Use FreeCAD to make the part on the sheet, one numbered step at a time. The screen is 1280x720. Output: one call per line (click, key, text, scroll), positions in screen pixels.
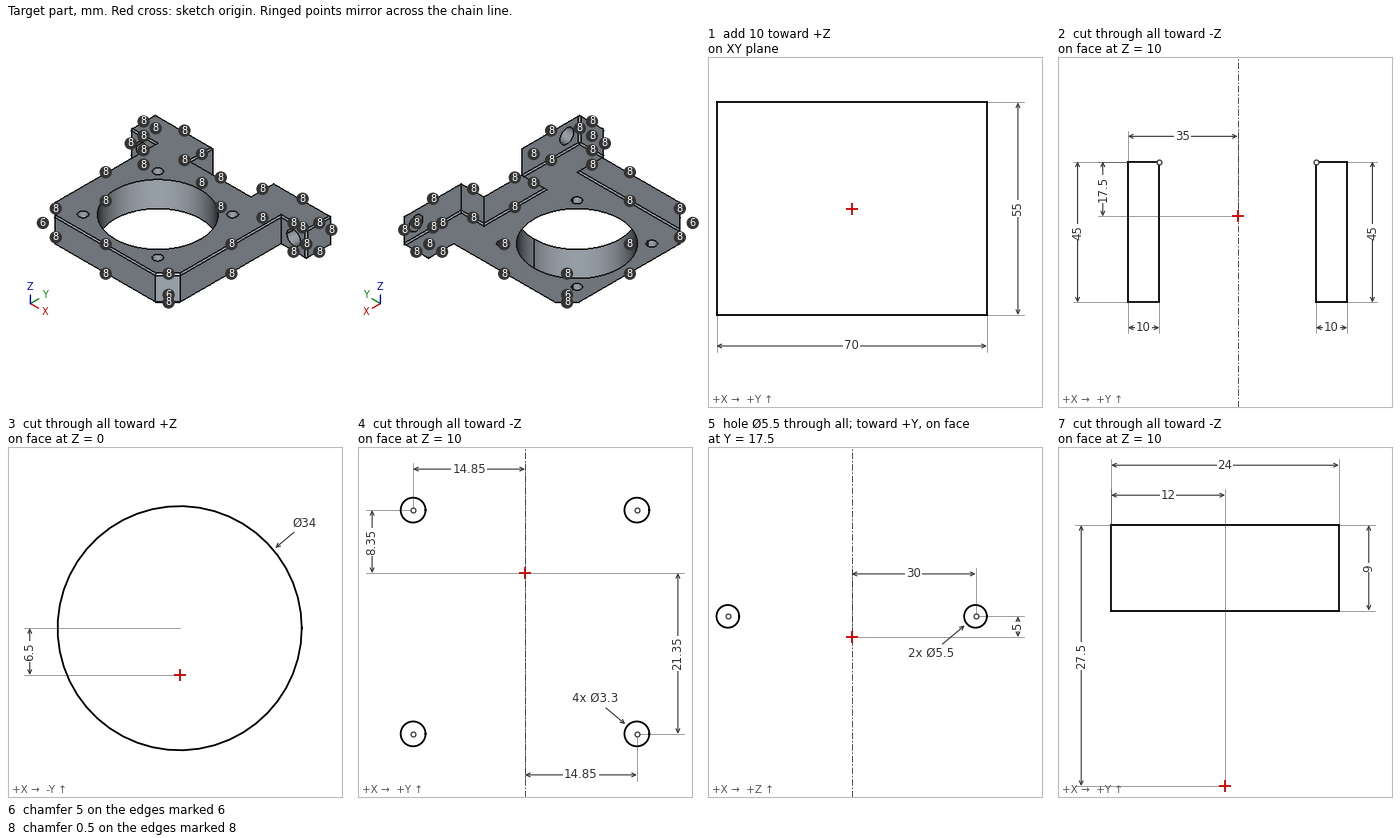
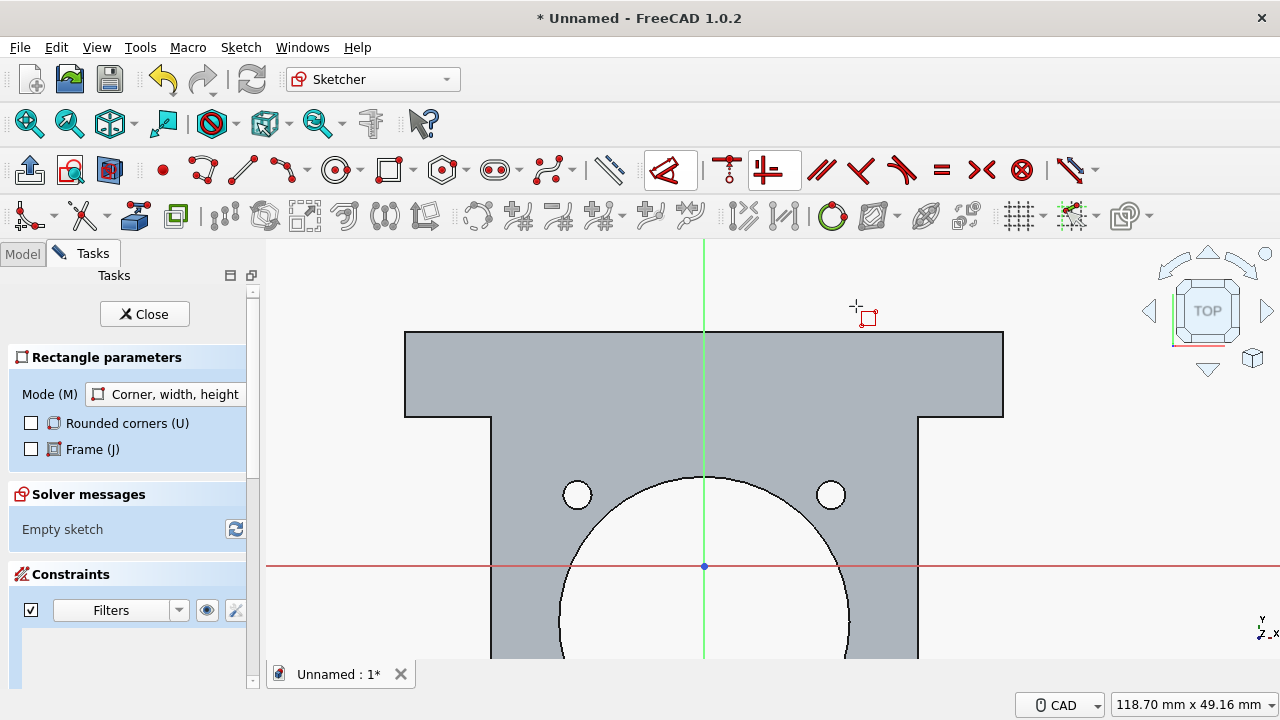
click(602, 332)
move(807, 408)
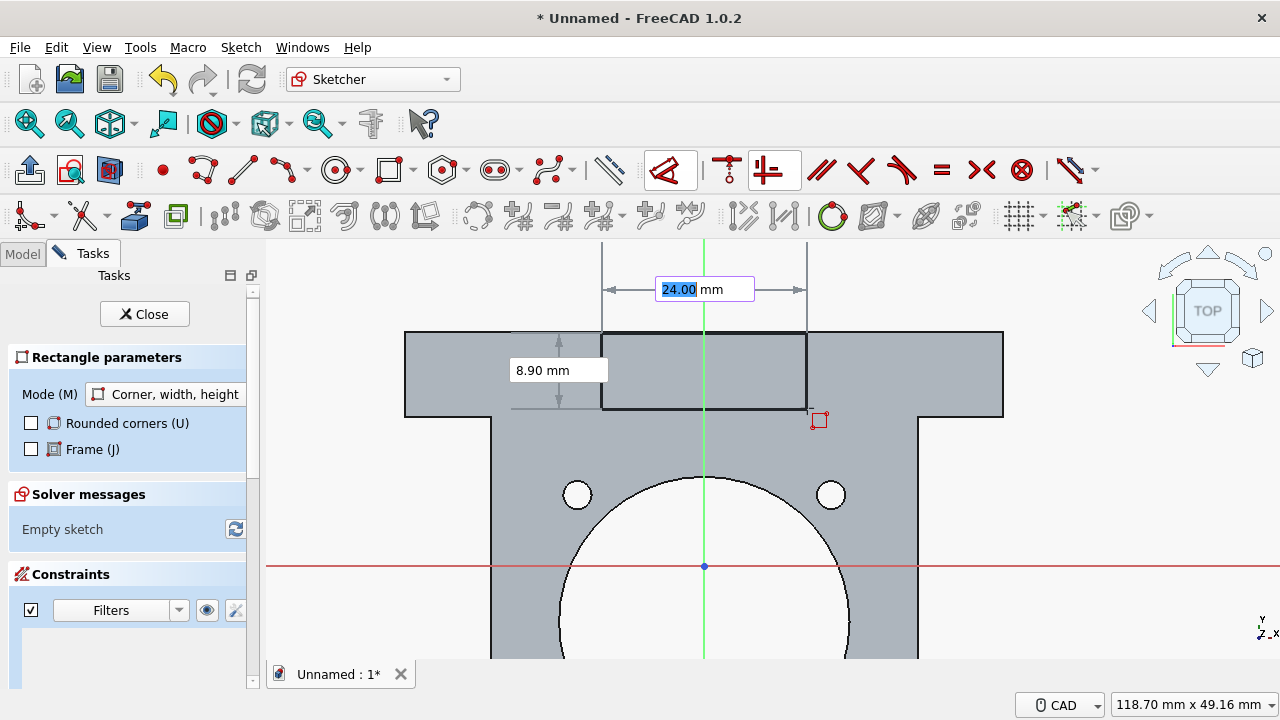
text(24)
key(Tab)
text(9)
key(Return)
key(Escape)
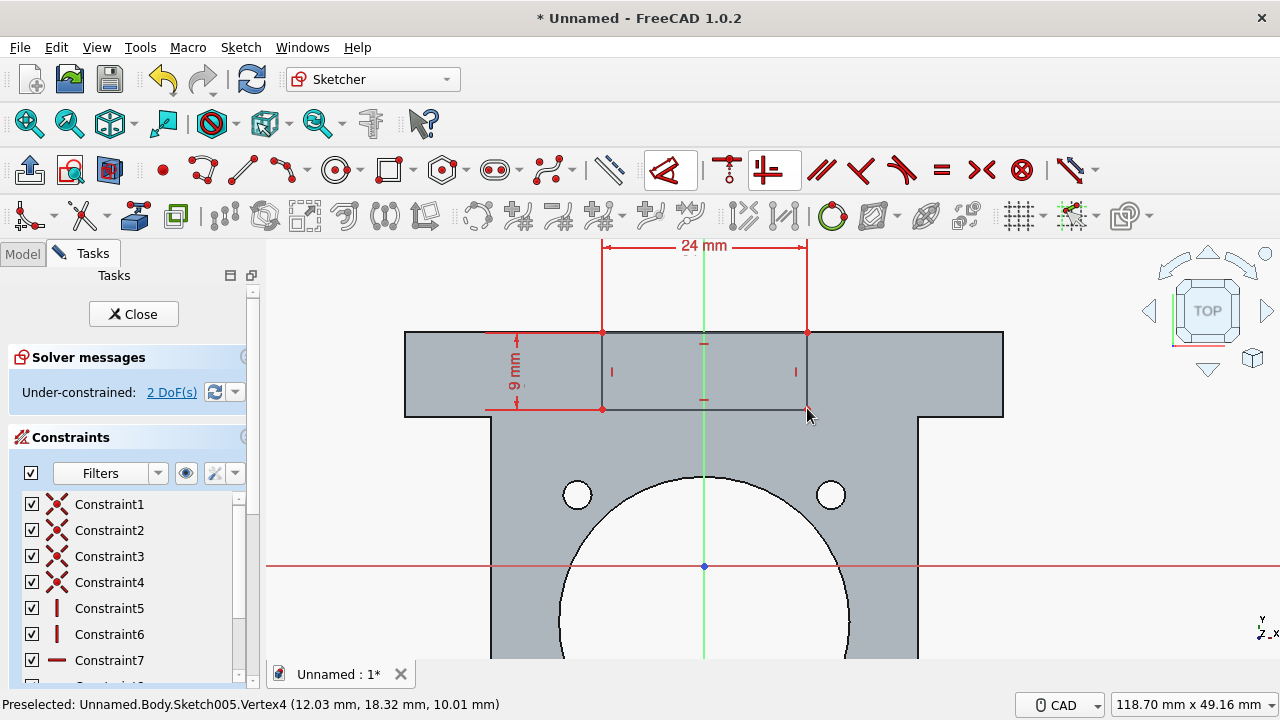
click(602, 333)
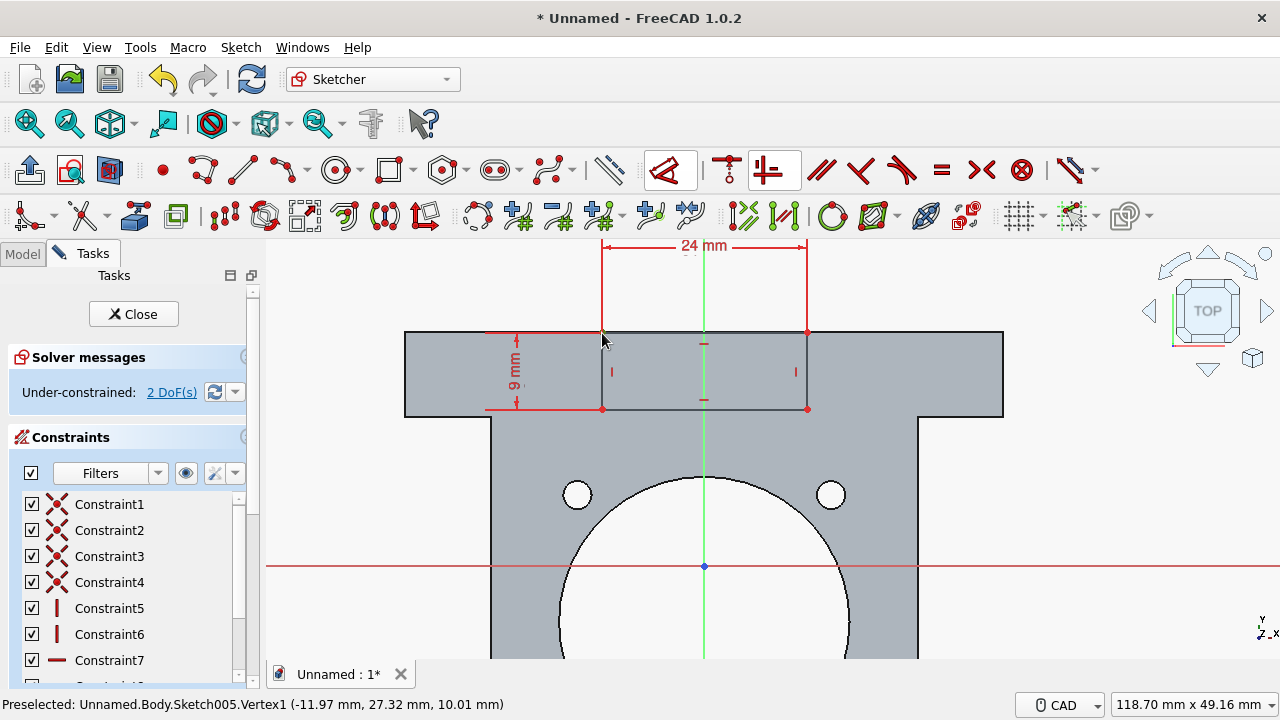
key(l)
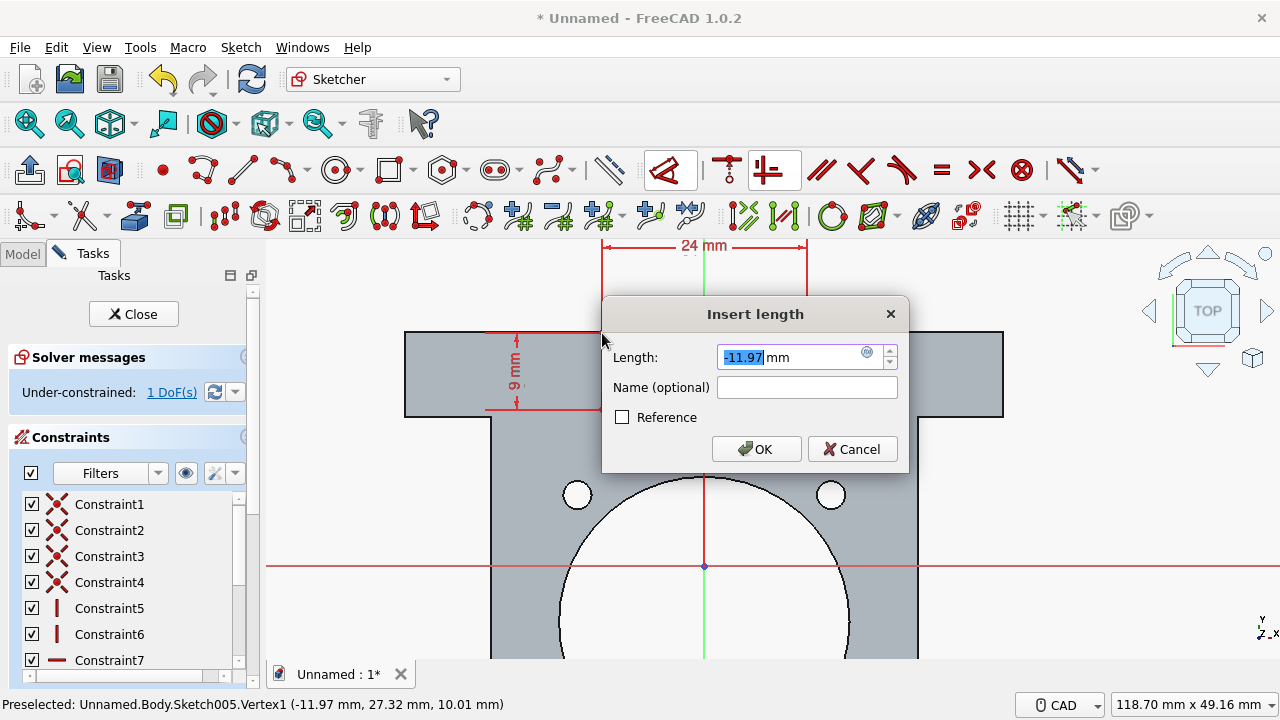
text(-12)
key(Return)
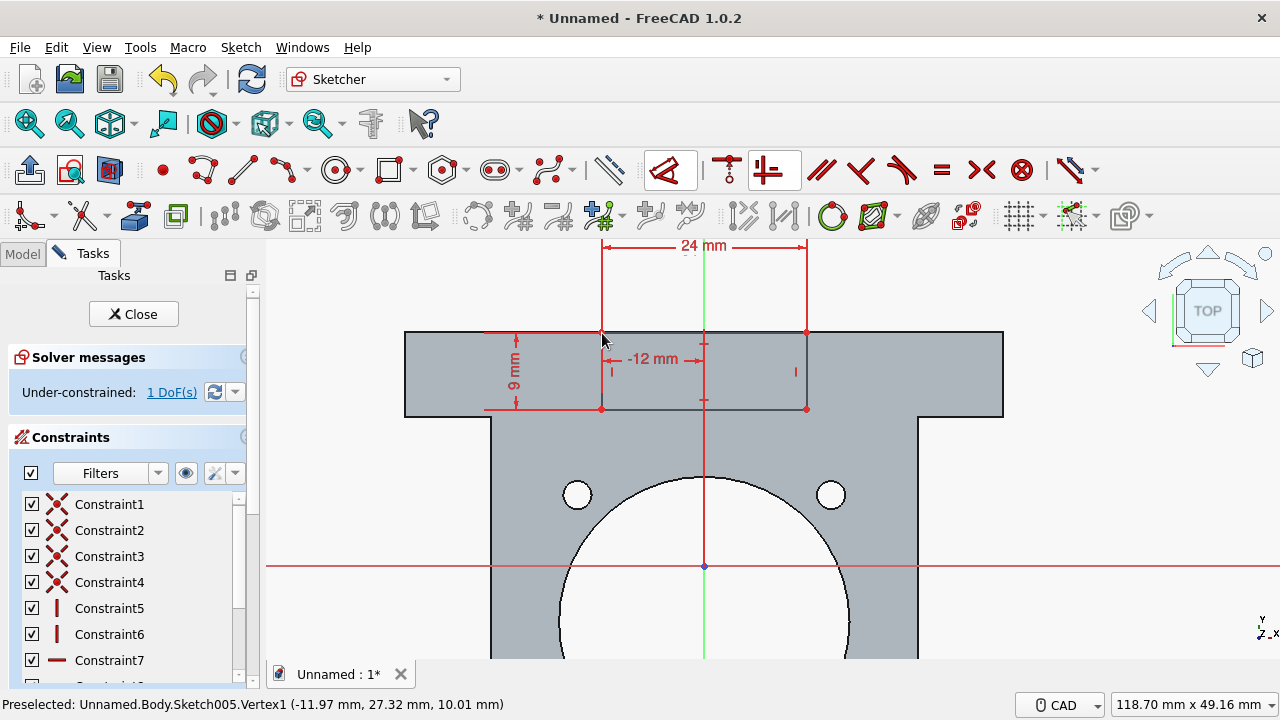
click(602, 333)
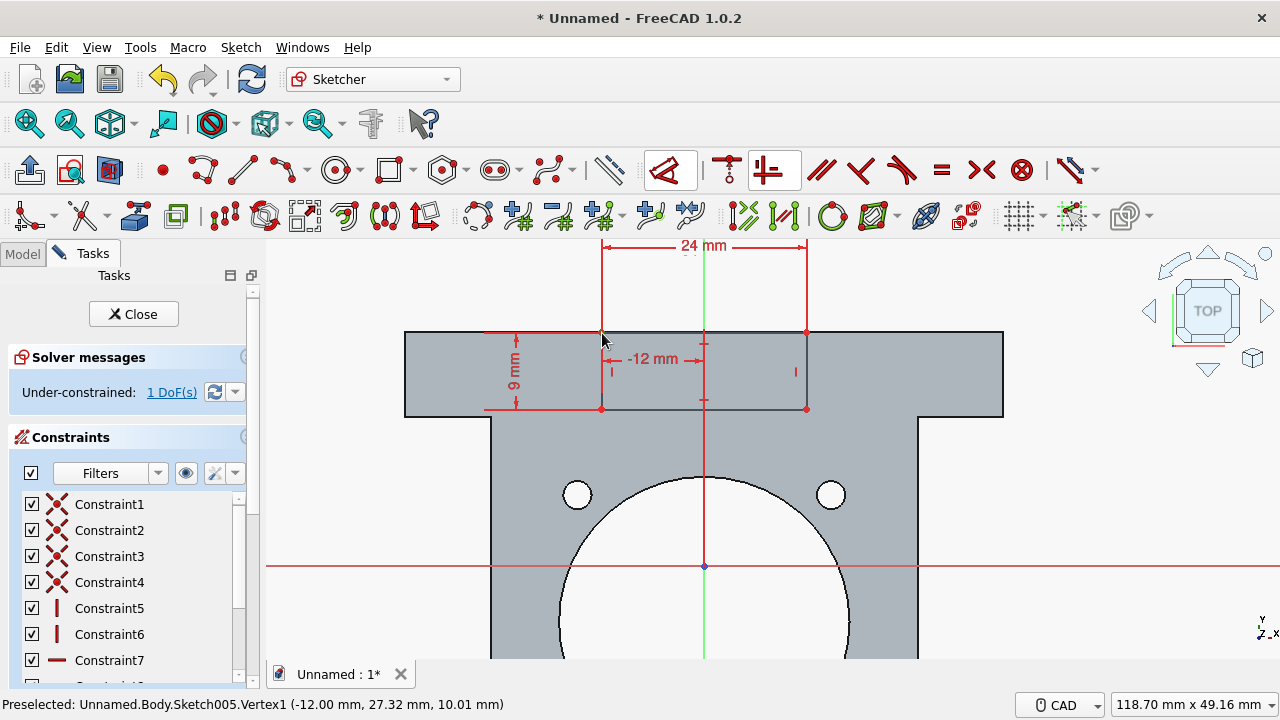
click(692, 170)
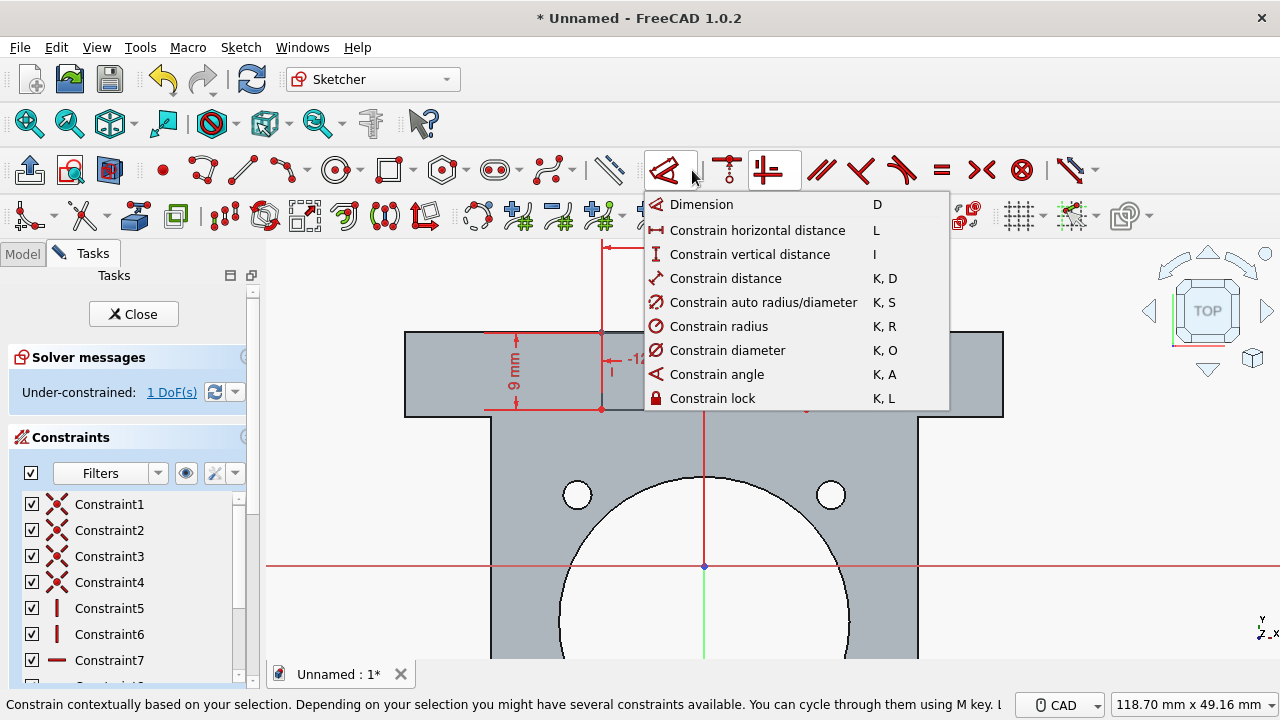
click(797, 254)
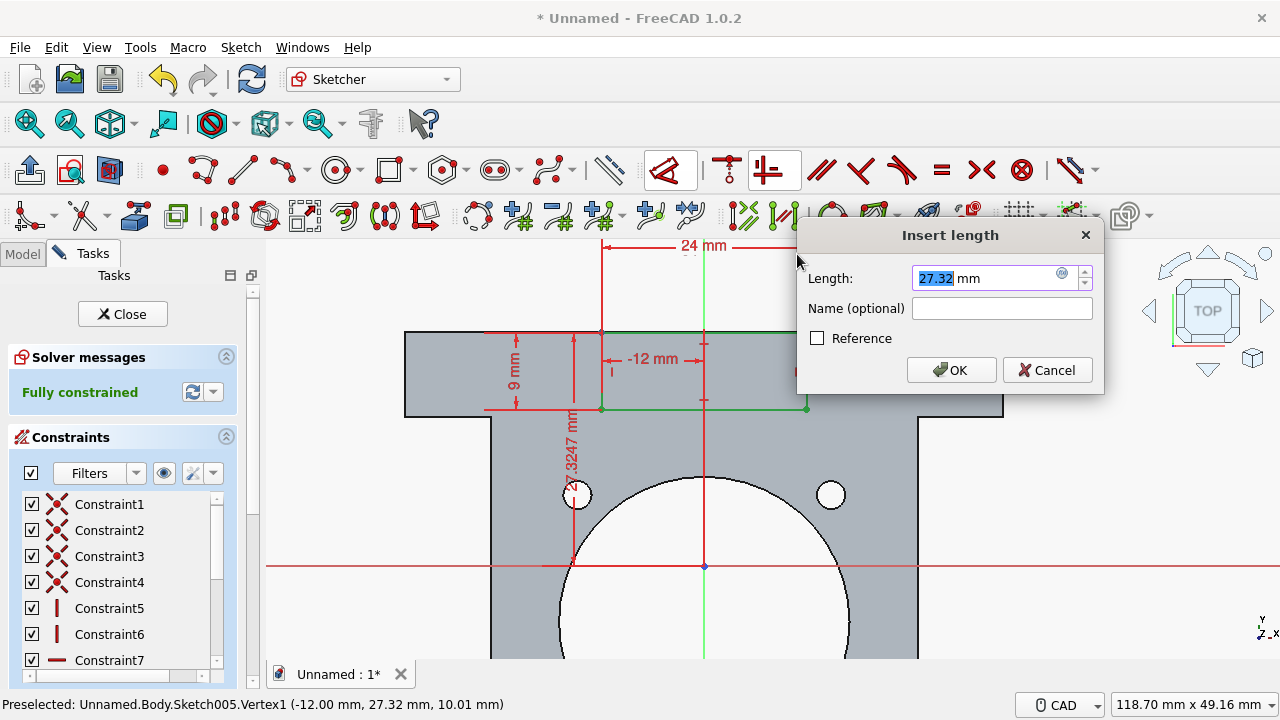
text(27.5)
key(Return)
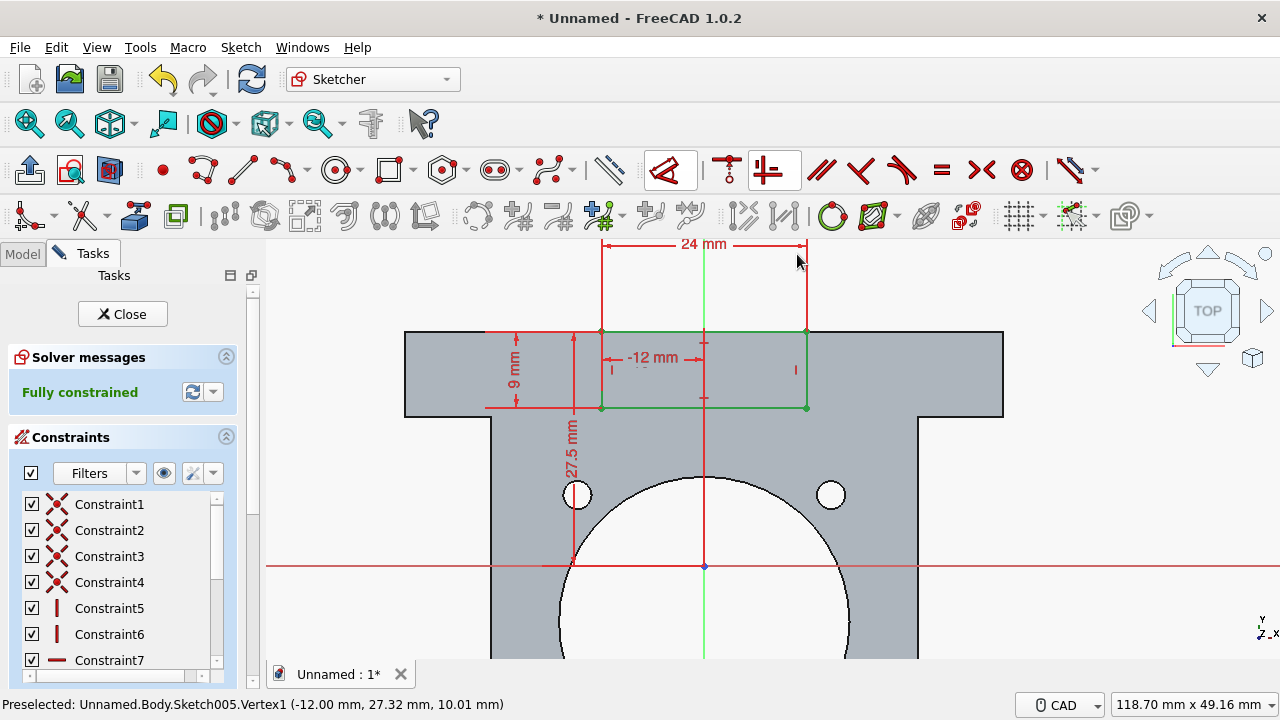
click(123, 314)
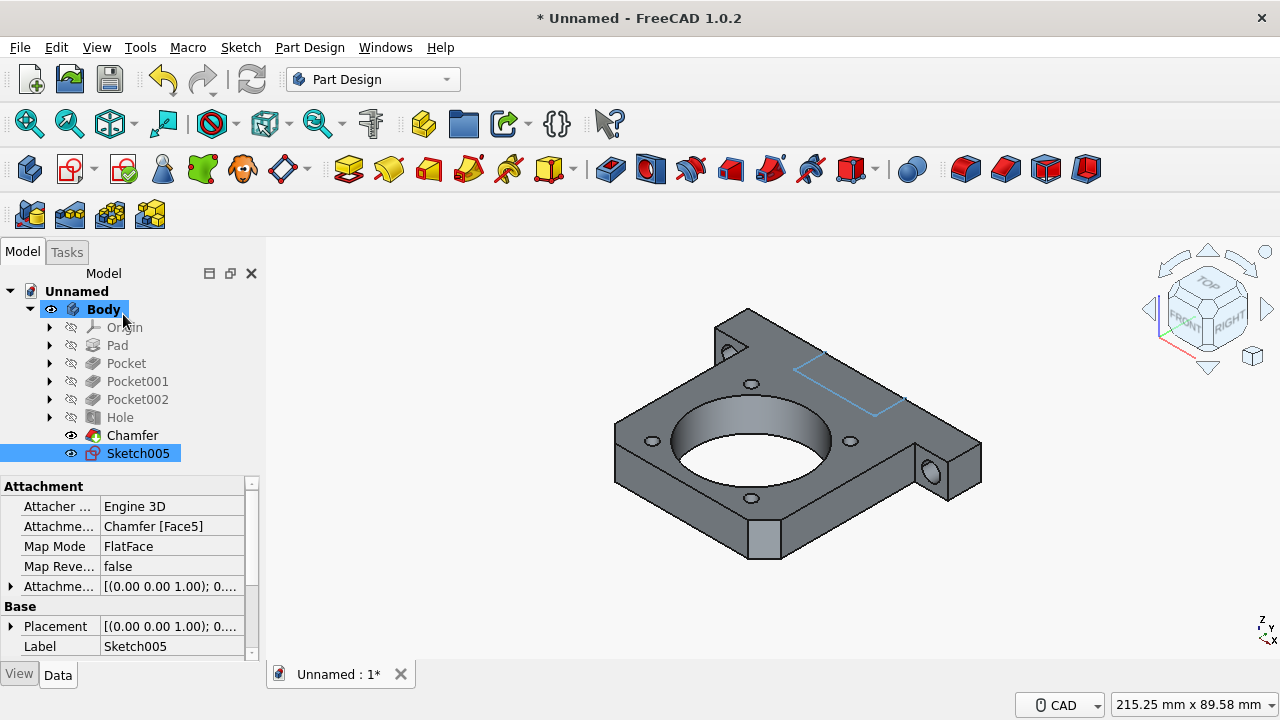
click(612, 170)